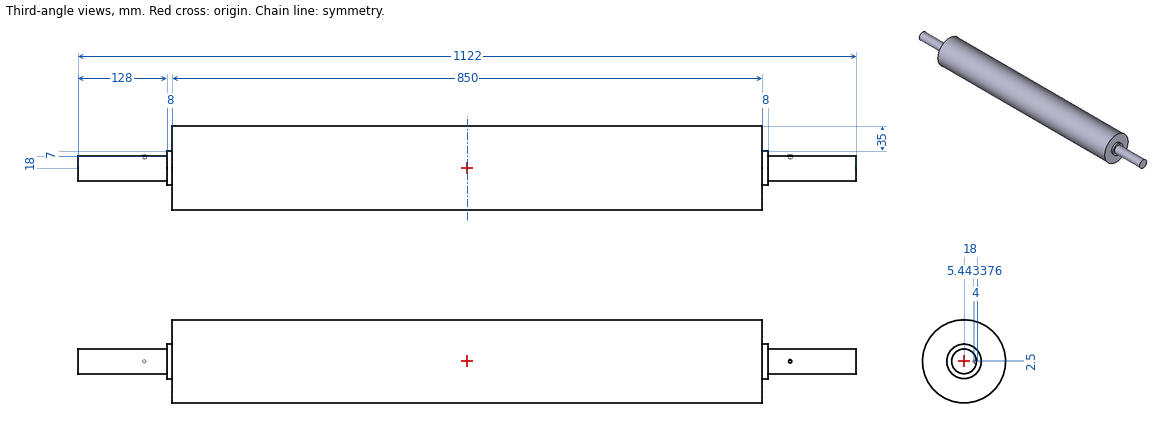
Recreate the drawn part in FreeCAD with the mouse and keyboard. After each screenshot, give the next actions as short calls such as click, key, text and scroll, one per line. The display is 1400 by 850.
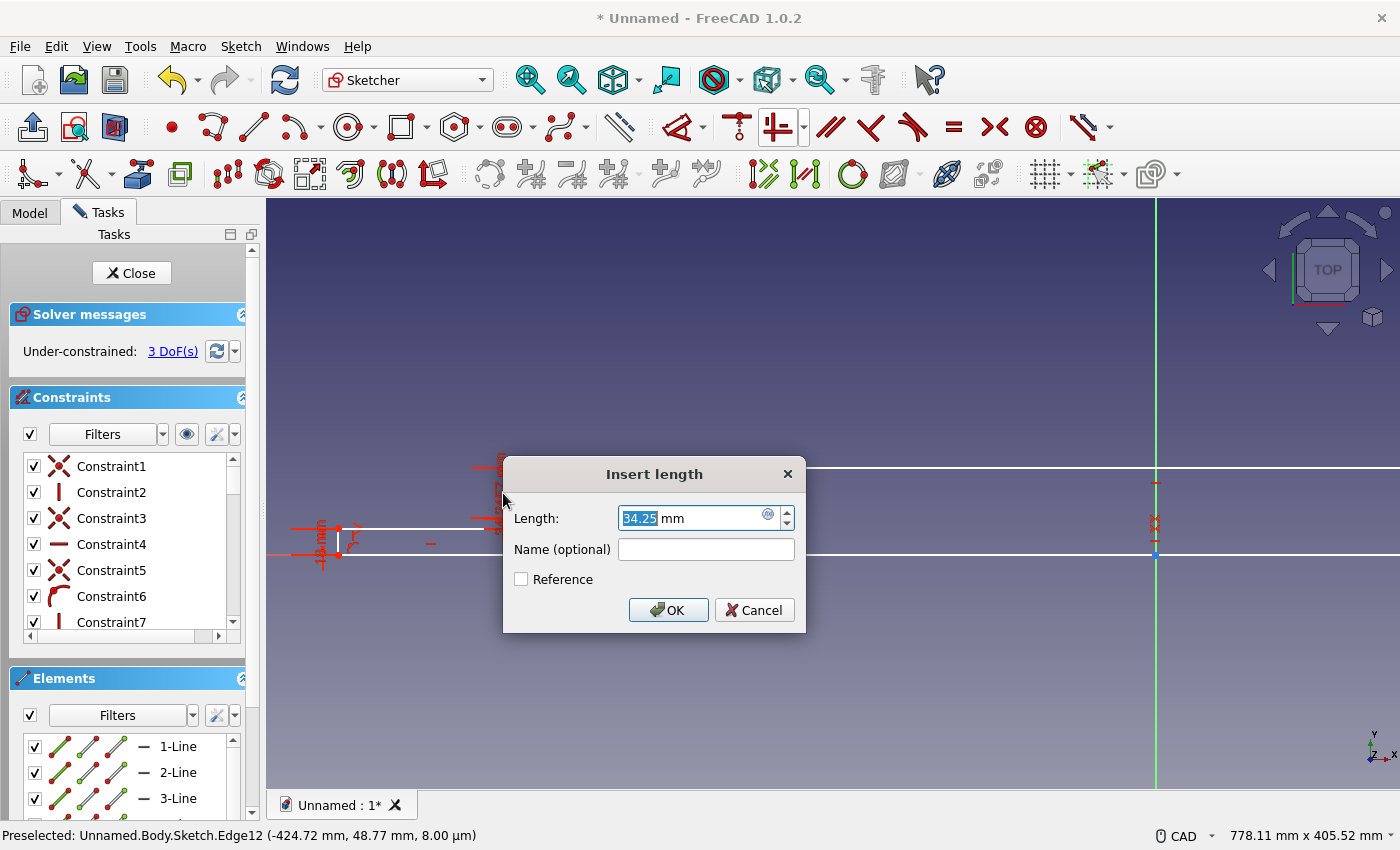
text(35)
key(Return)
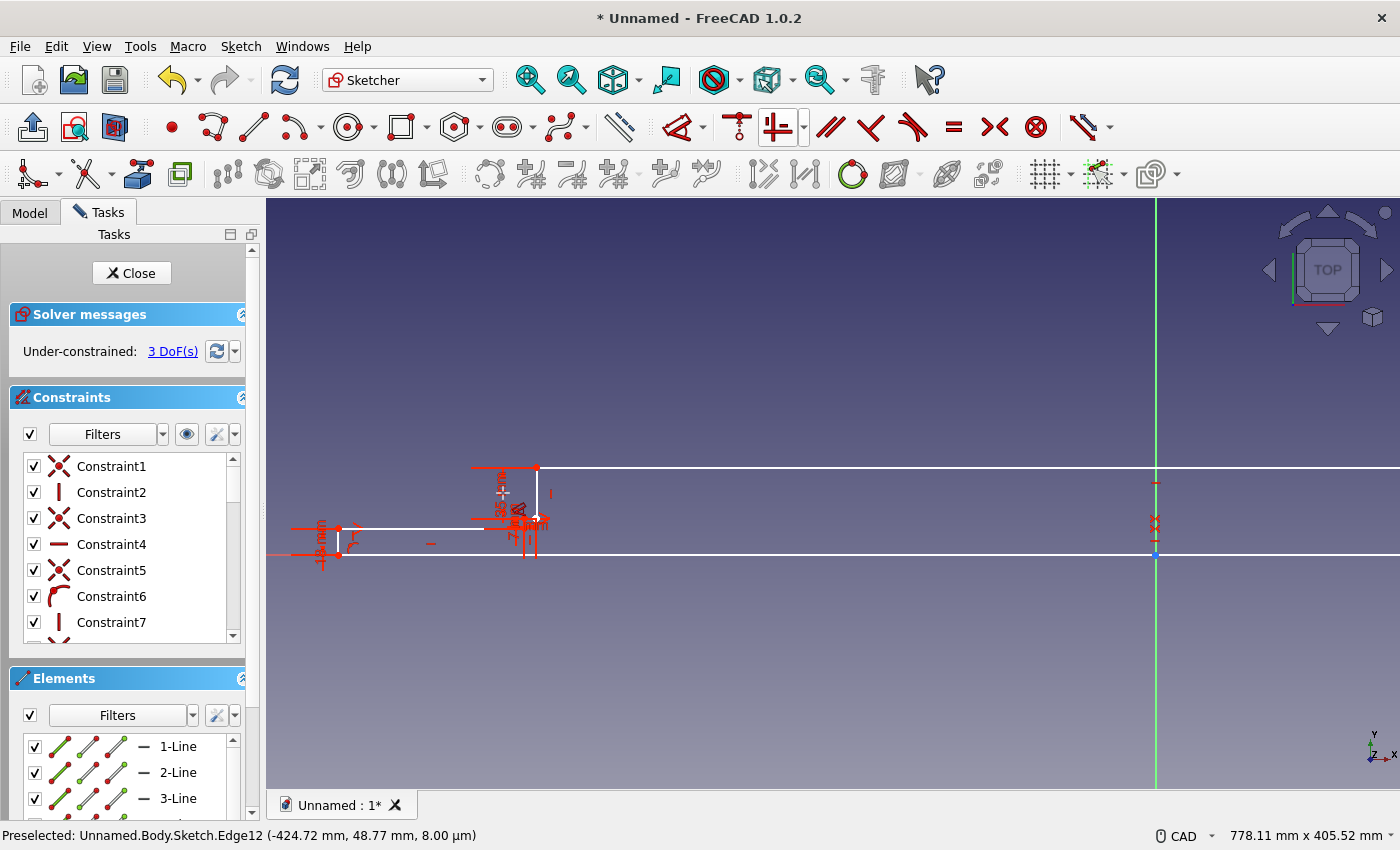
click(468, 529)
click(431, 495)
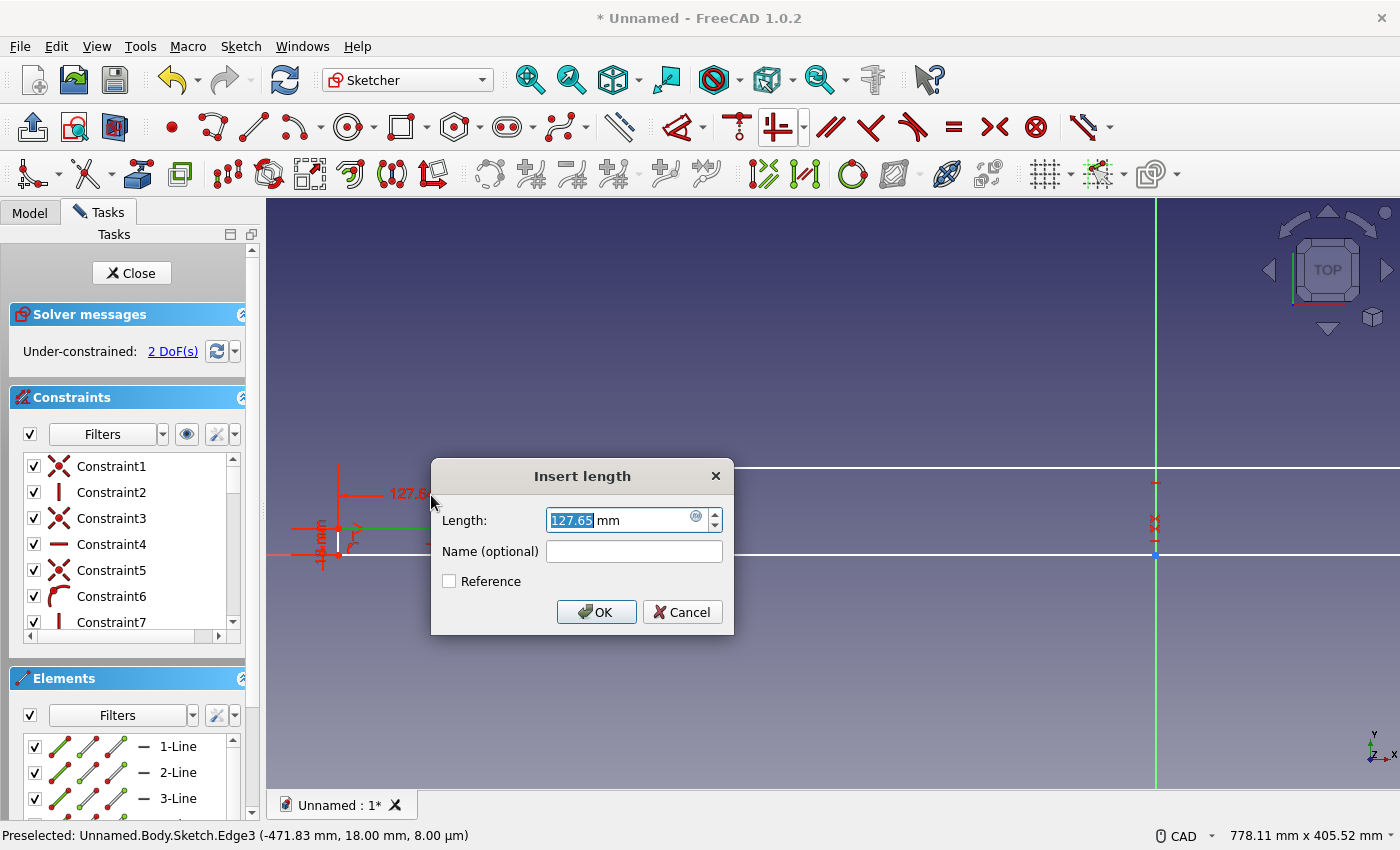
text(128)
key(Return)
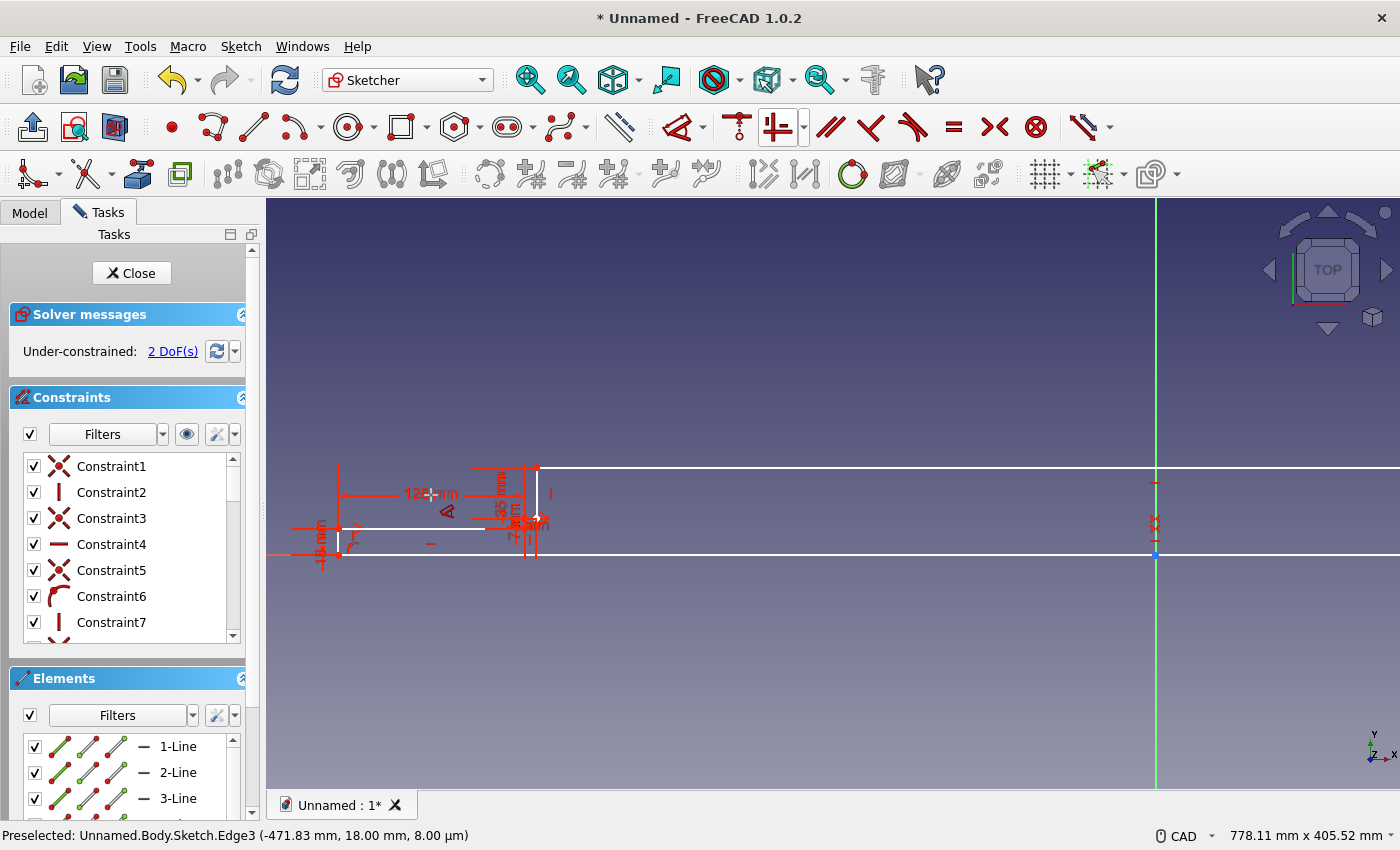
click(908, 468)
click(886, 434)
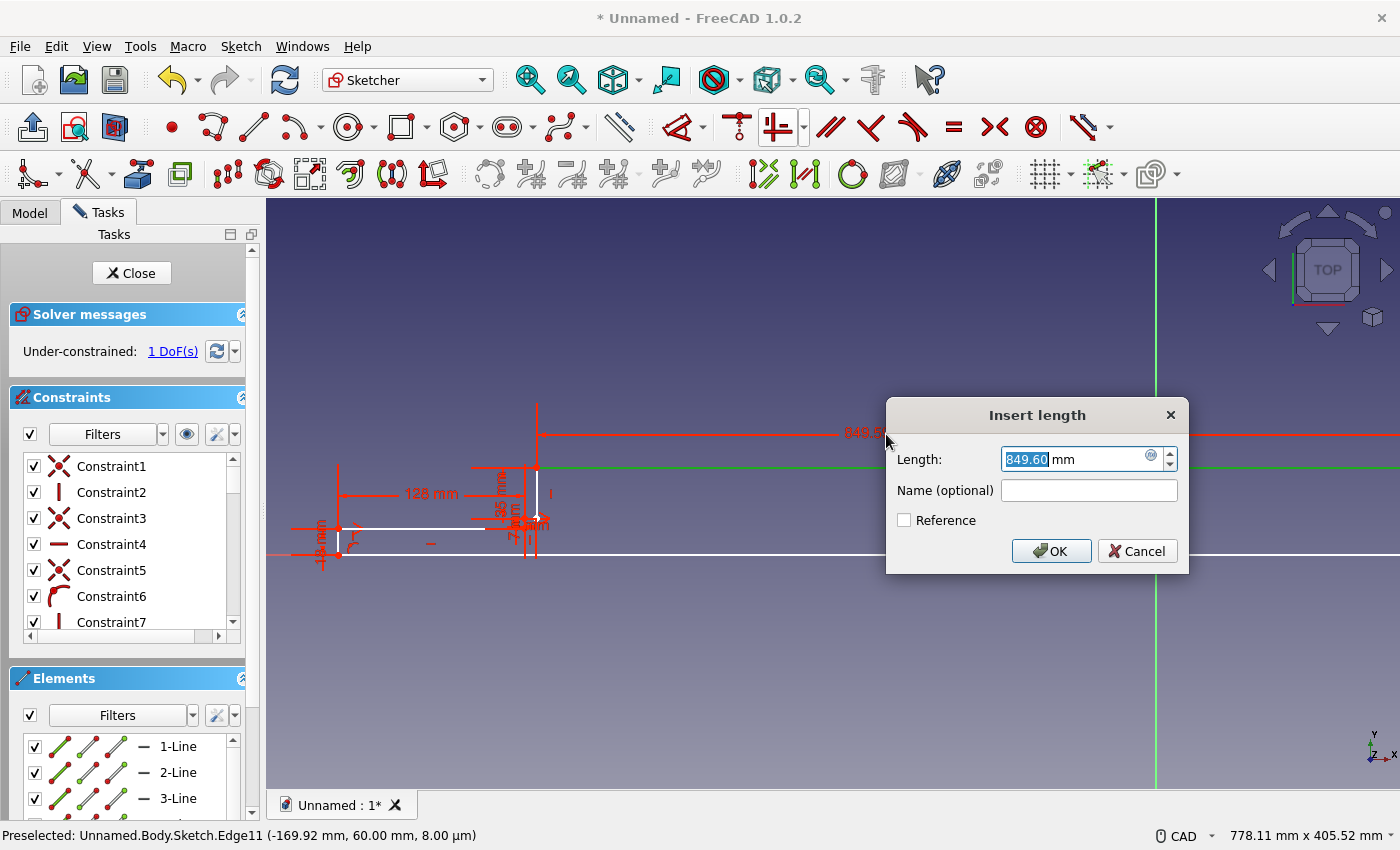
text(850)
key(Return)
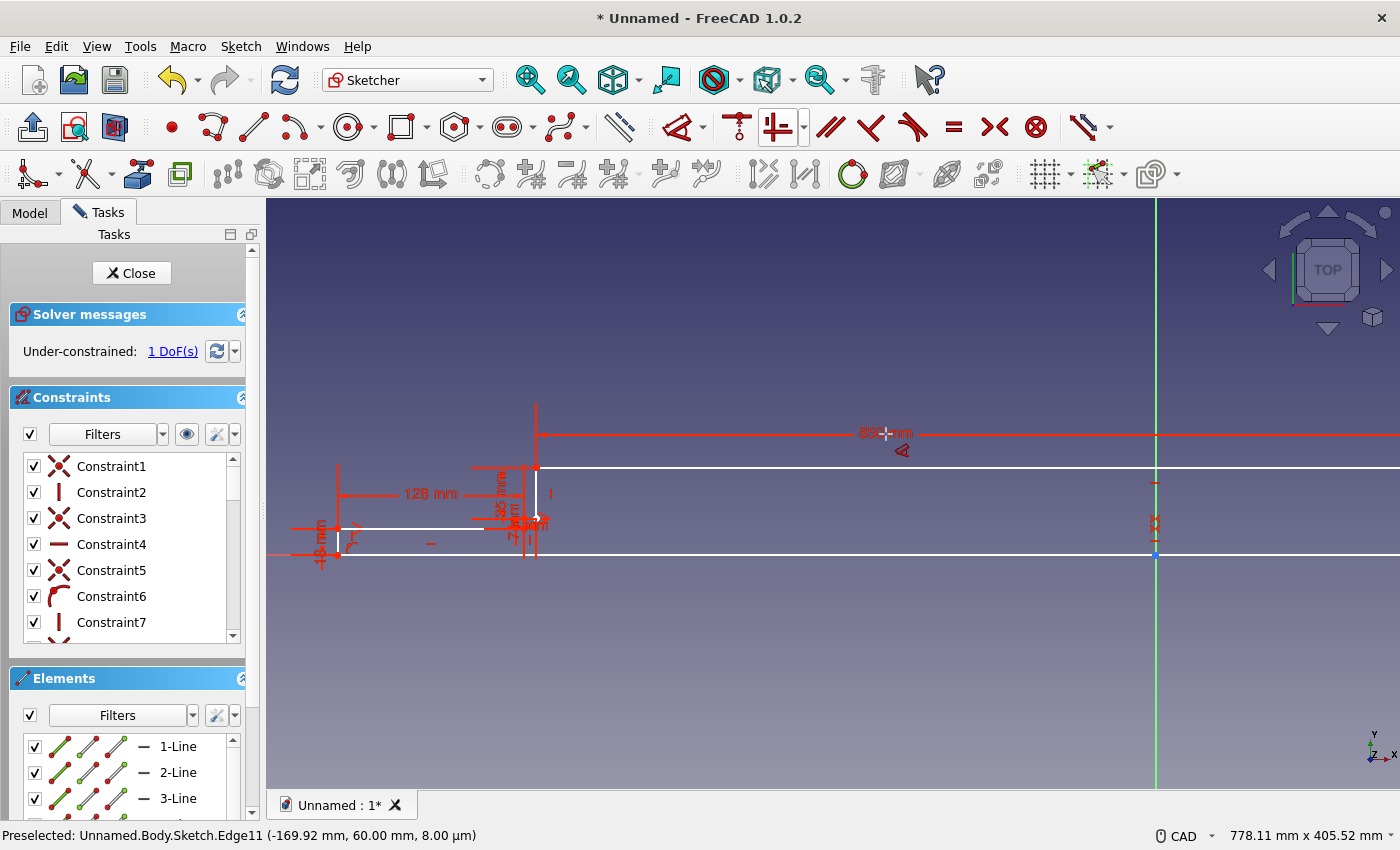
click(829, 555)
click(786, 589)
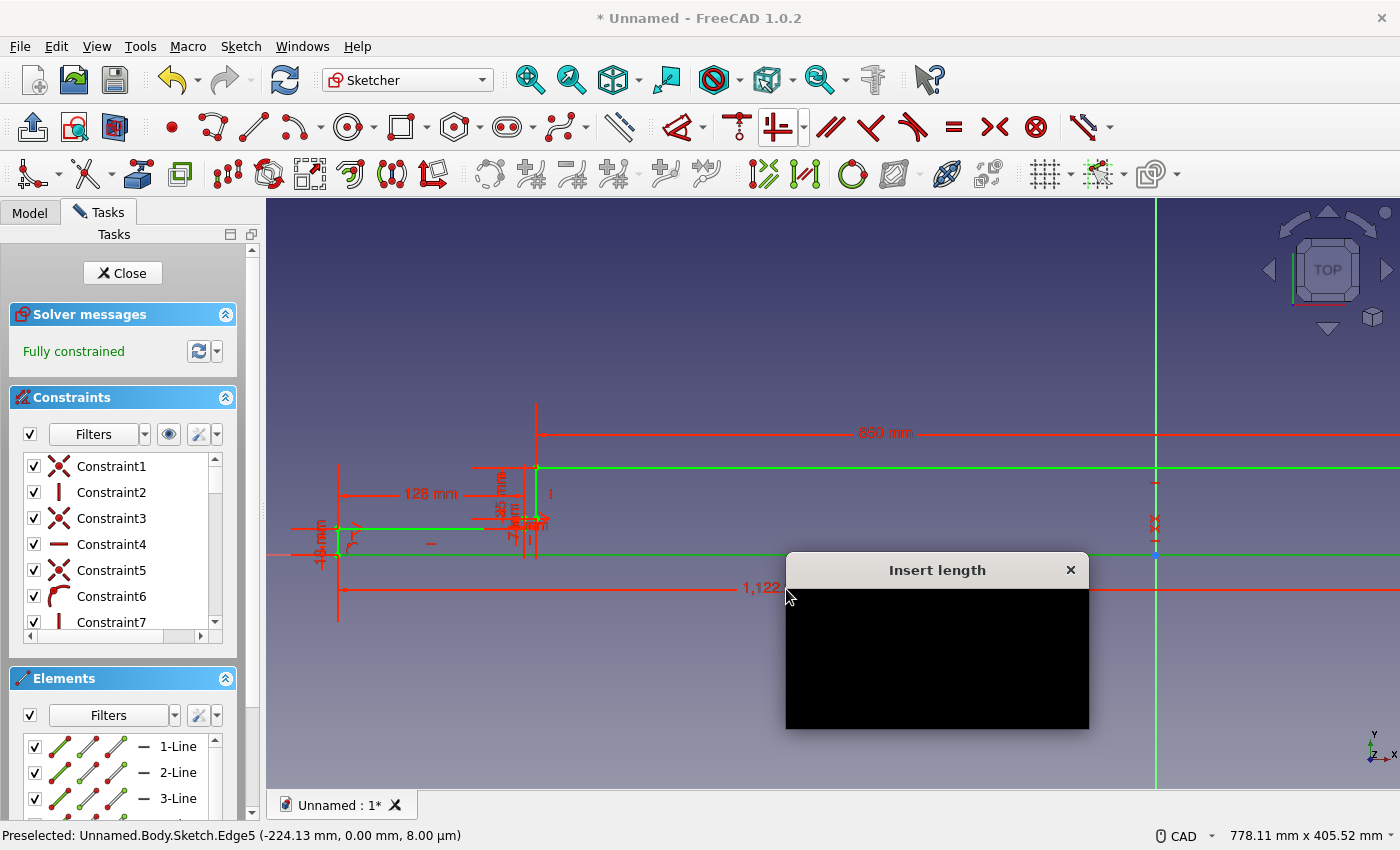
text(1122)
key(Return)
key(Escape)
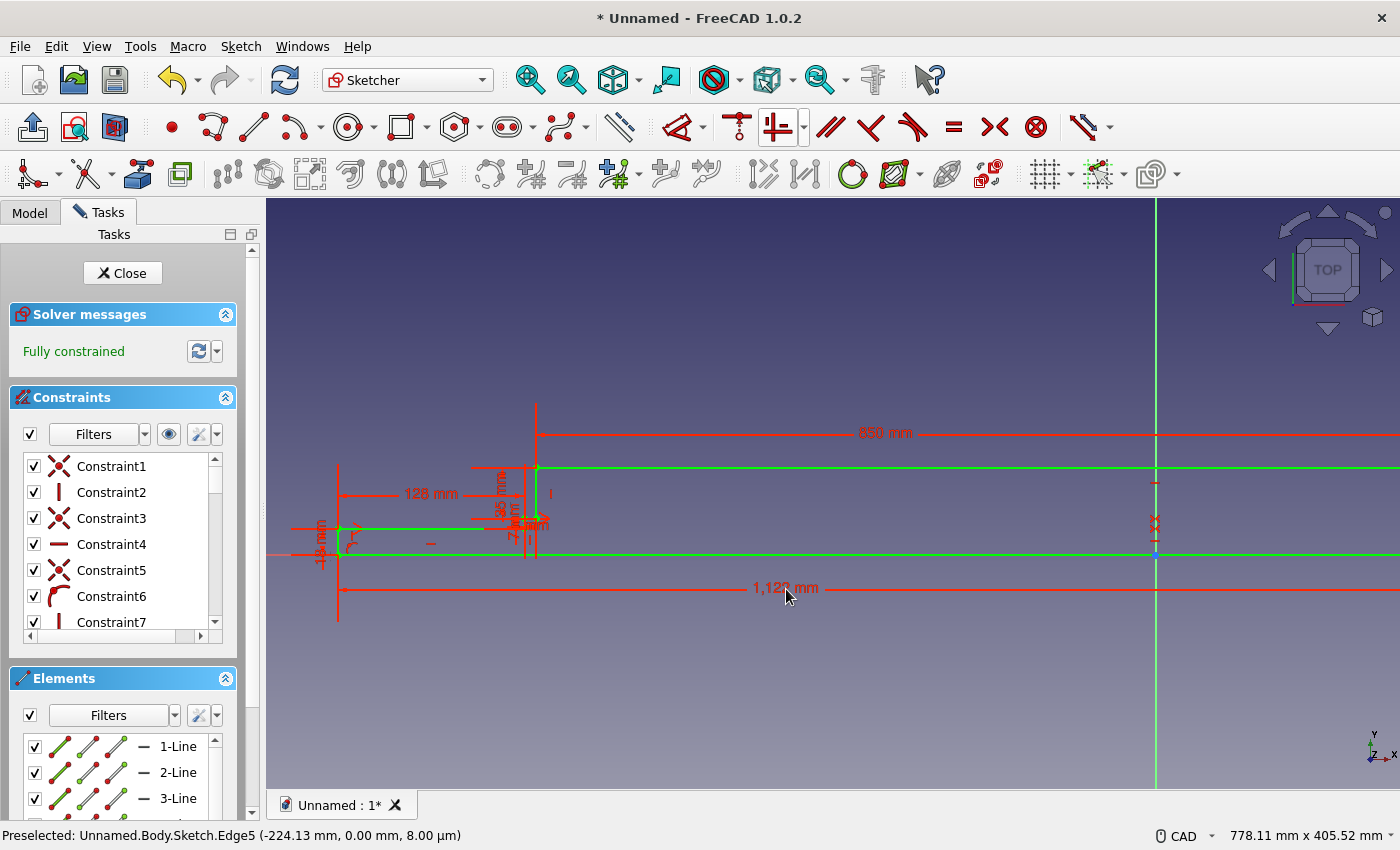
click(123, 273)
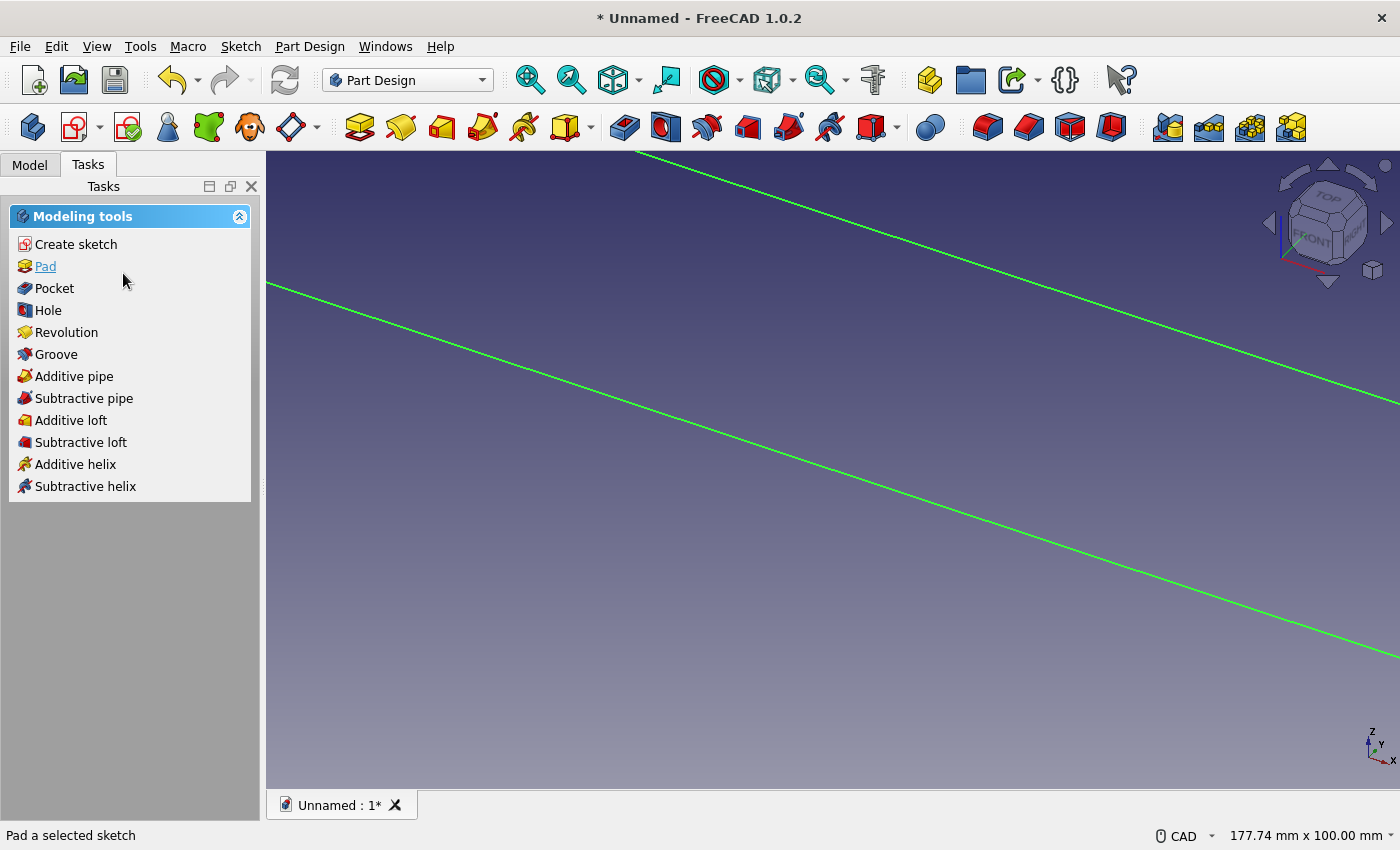
click(401, 128)